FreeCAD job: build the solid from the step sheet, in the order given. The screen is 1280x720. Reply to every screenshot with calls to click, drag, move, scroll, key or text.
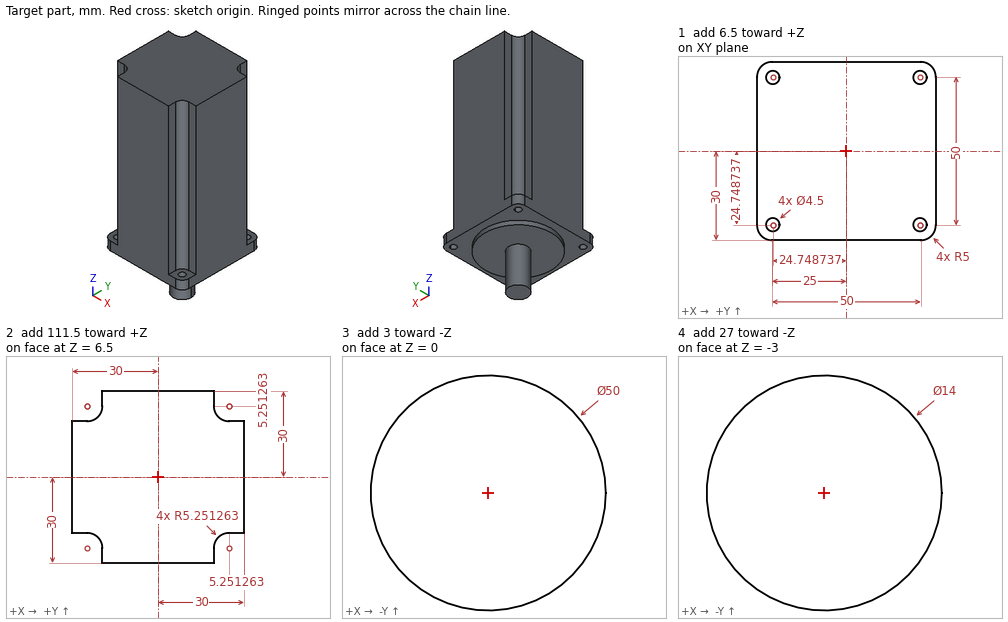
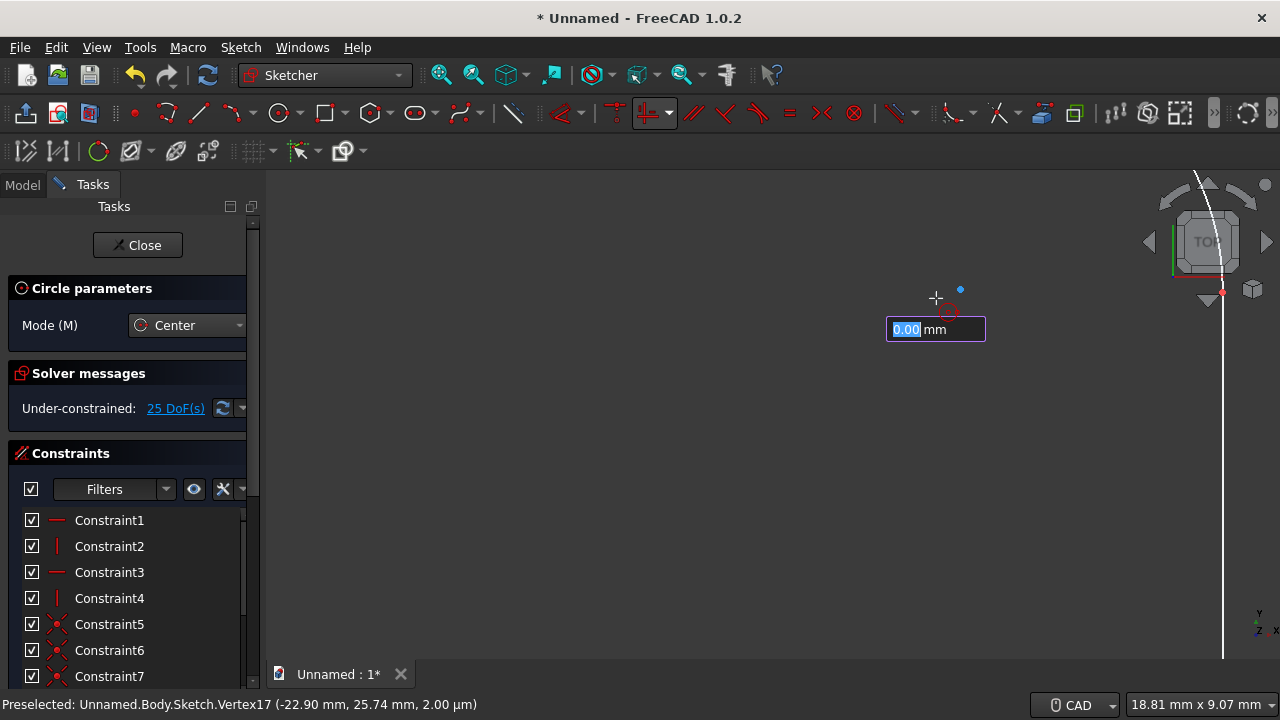
scroll(814, 293, down, 12)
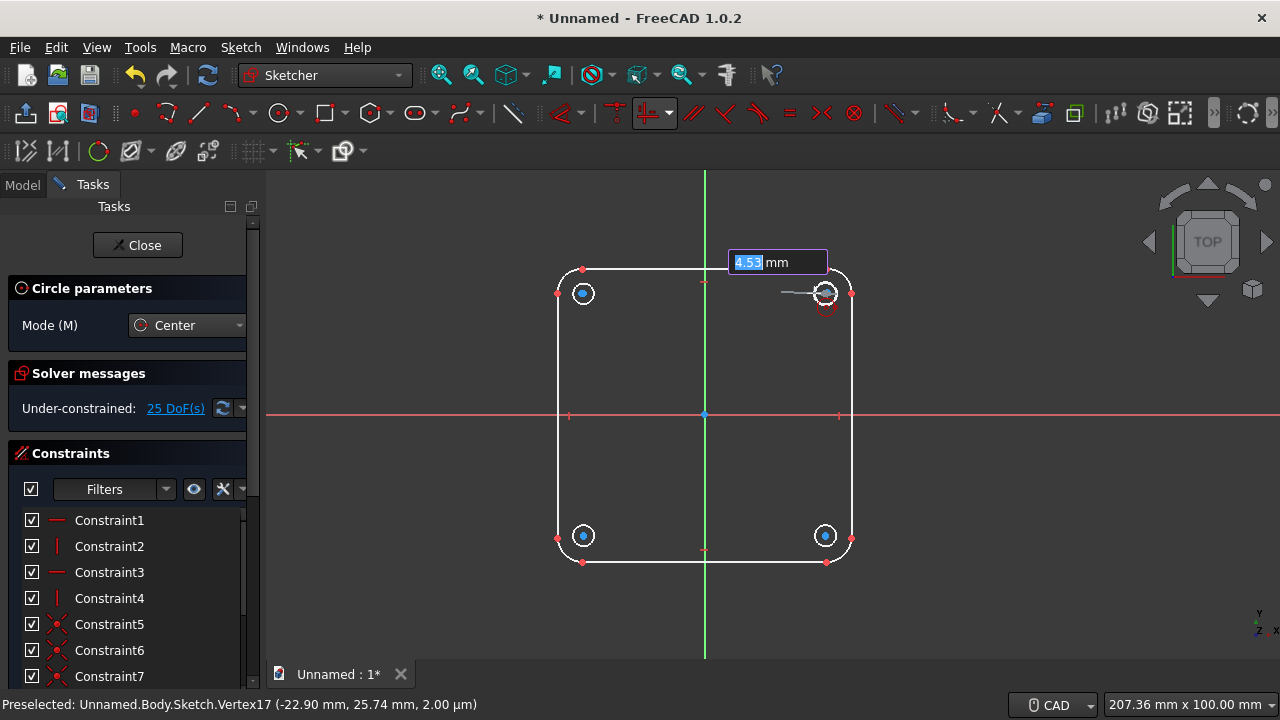
scroll(833, 286, up, 3)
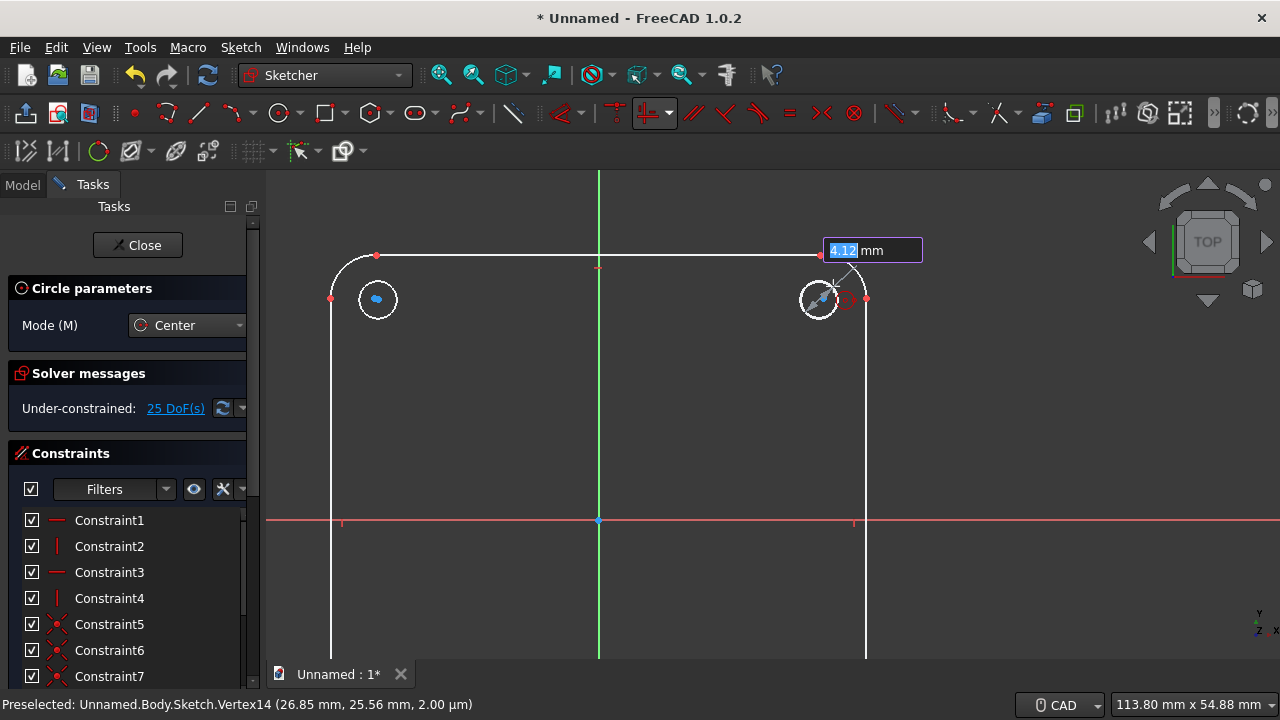
click(833, 286)
key(Escape)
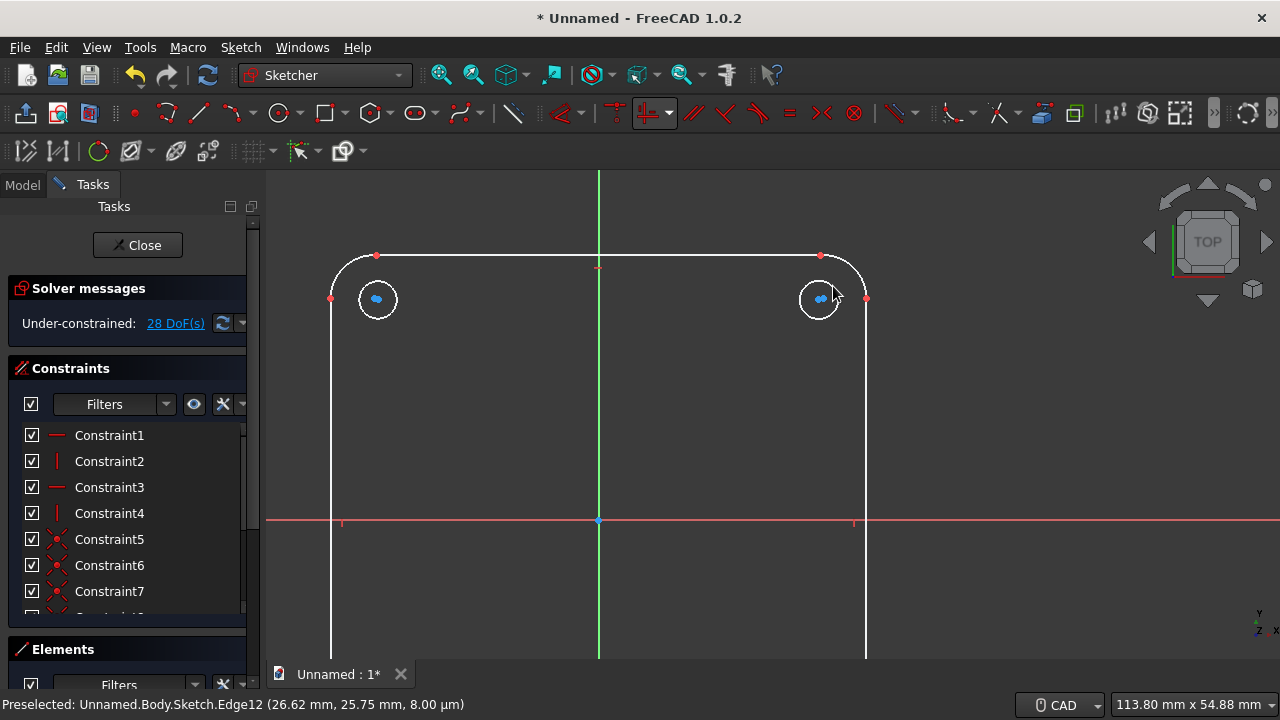
scroll(833, 286, down, 3)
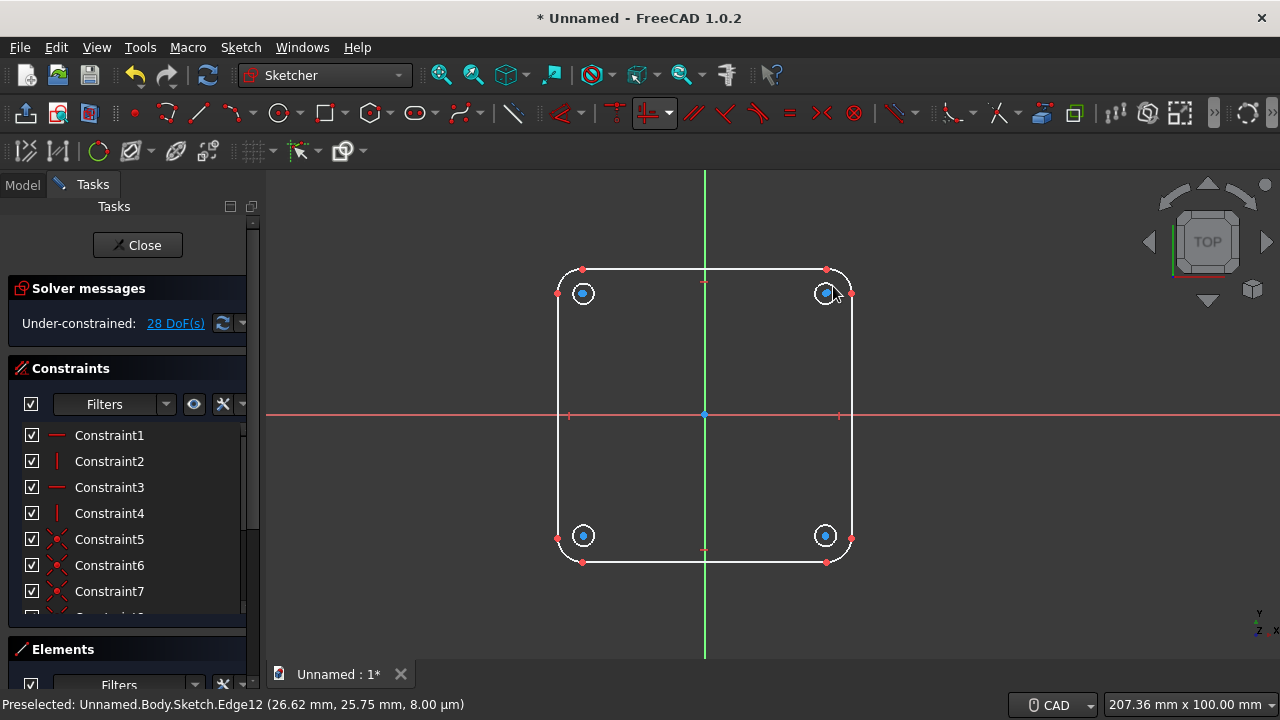
click(656, 562)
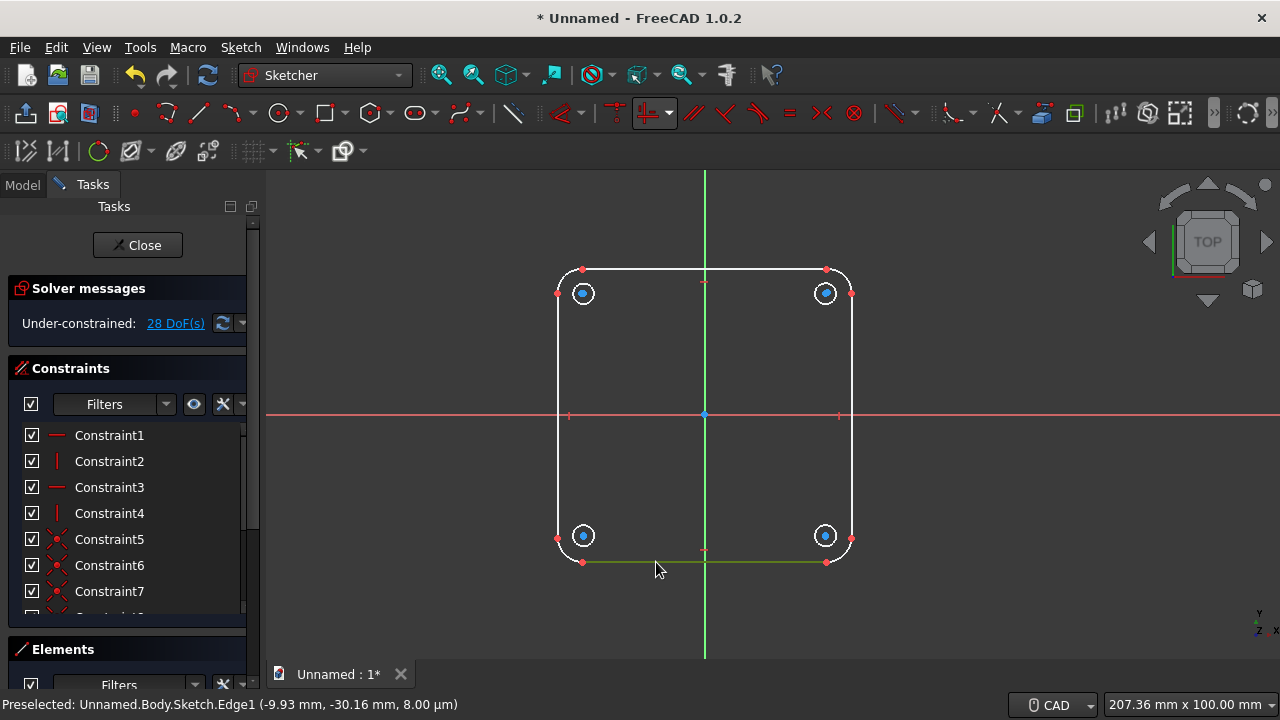
scroll(837, 559, up, 2)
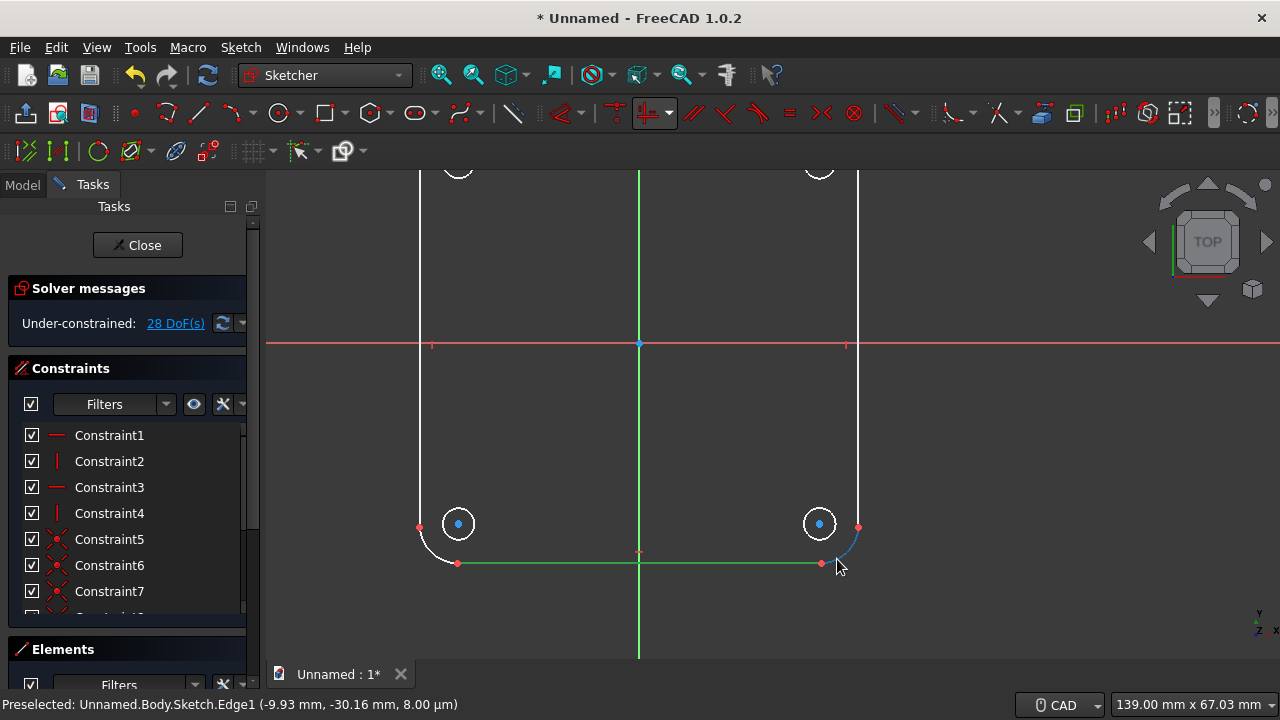
click(837, 559)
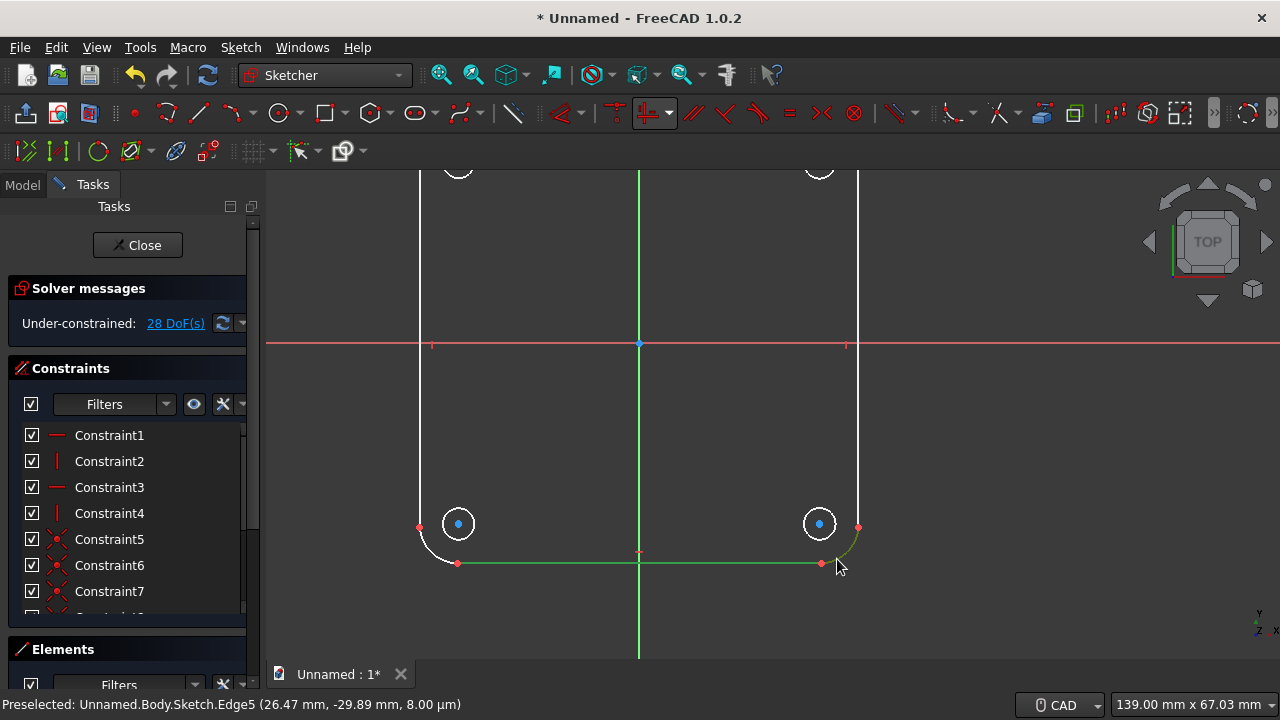
key(t)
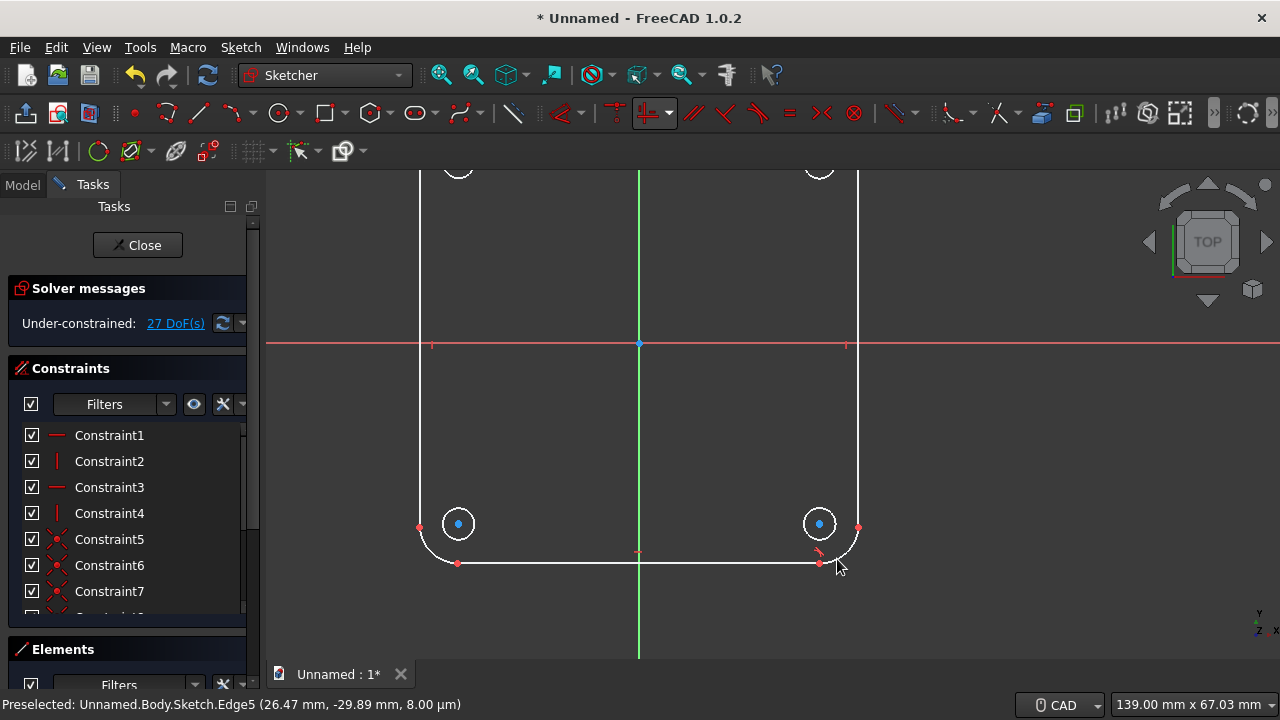
click(566, 563)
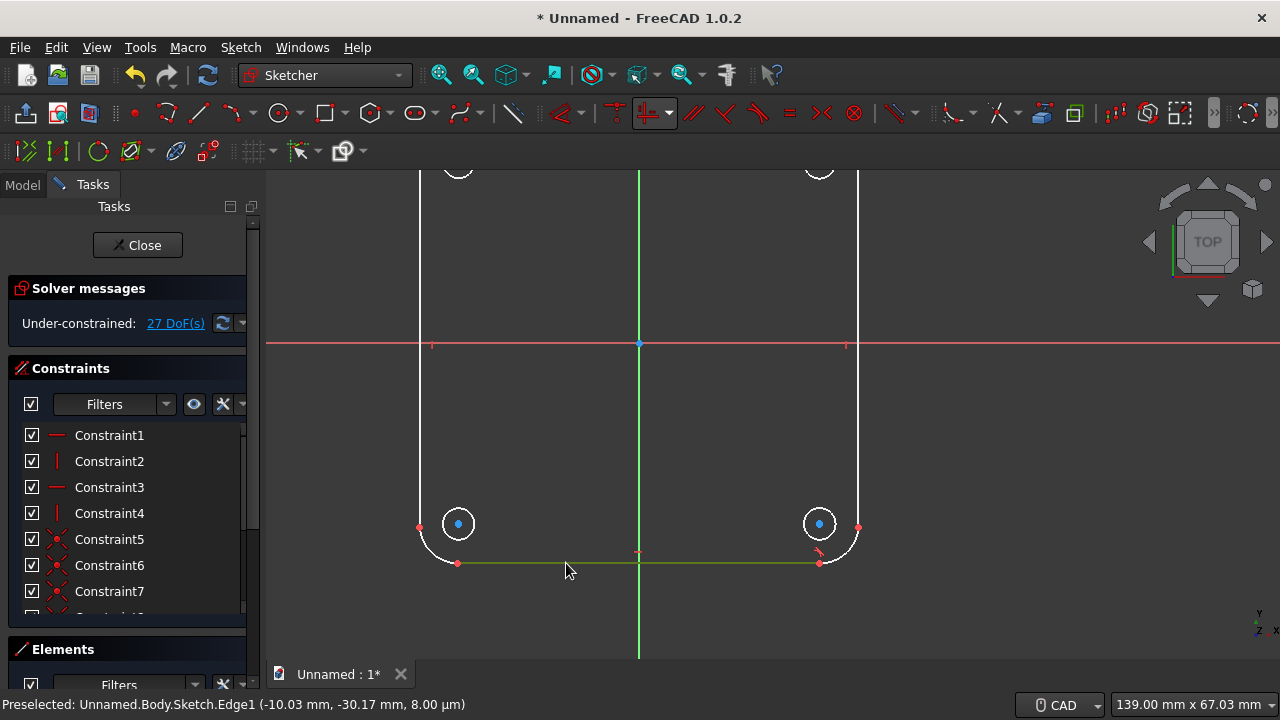
click(425, 544)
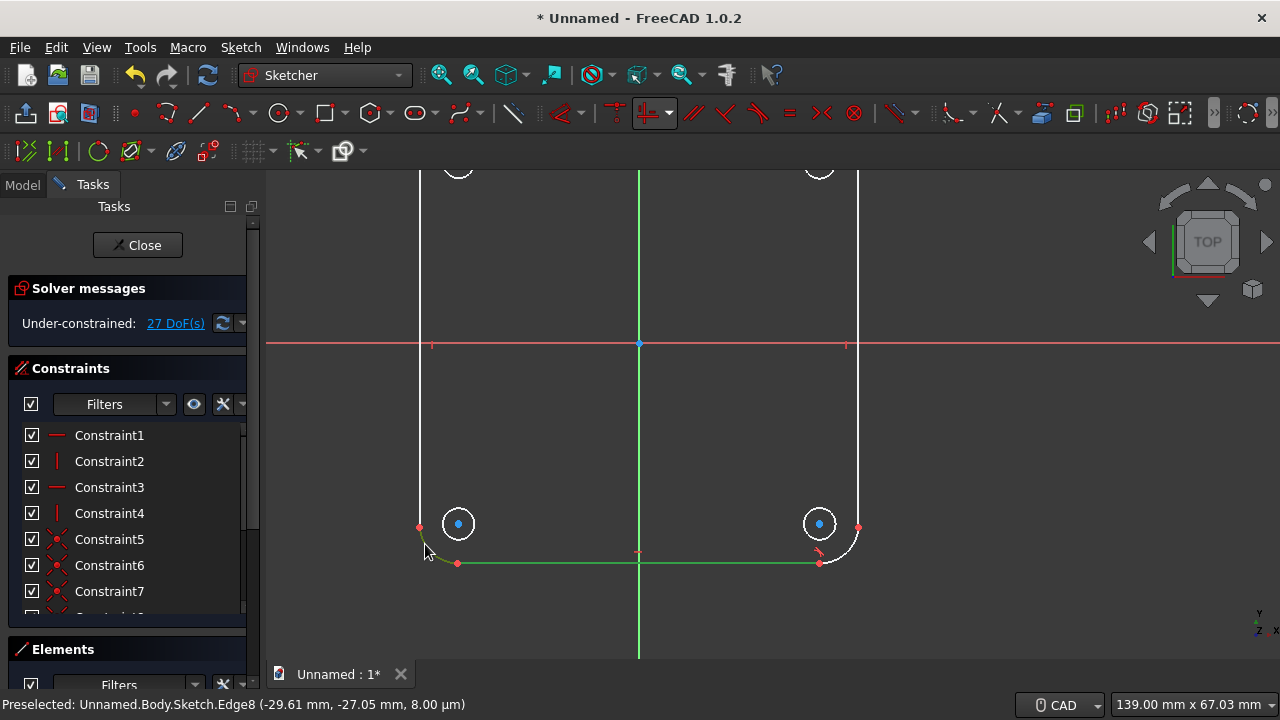
key(t)